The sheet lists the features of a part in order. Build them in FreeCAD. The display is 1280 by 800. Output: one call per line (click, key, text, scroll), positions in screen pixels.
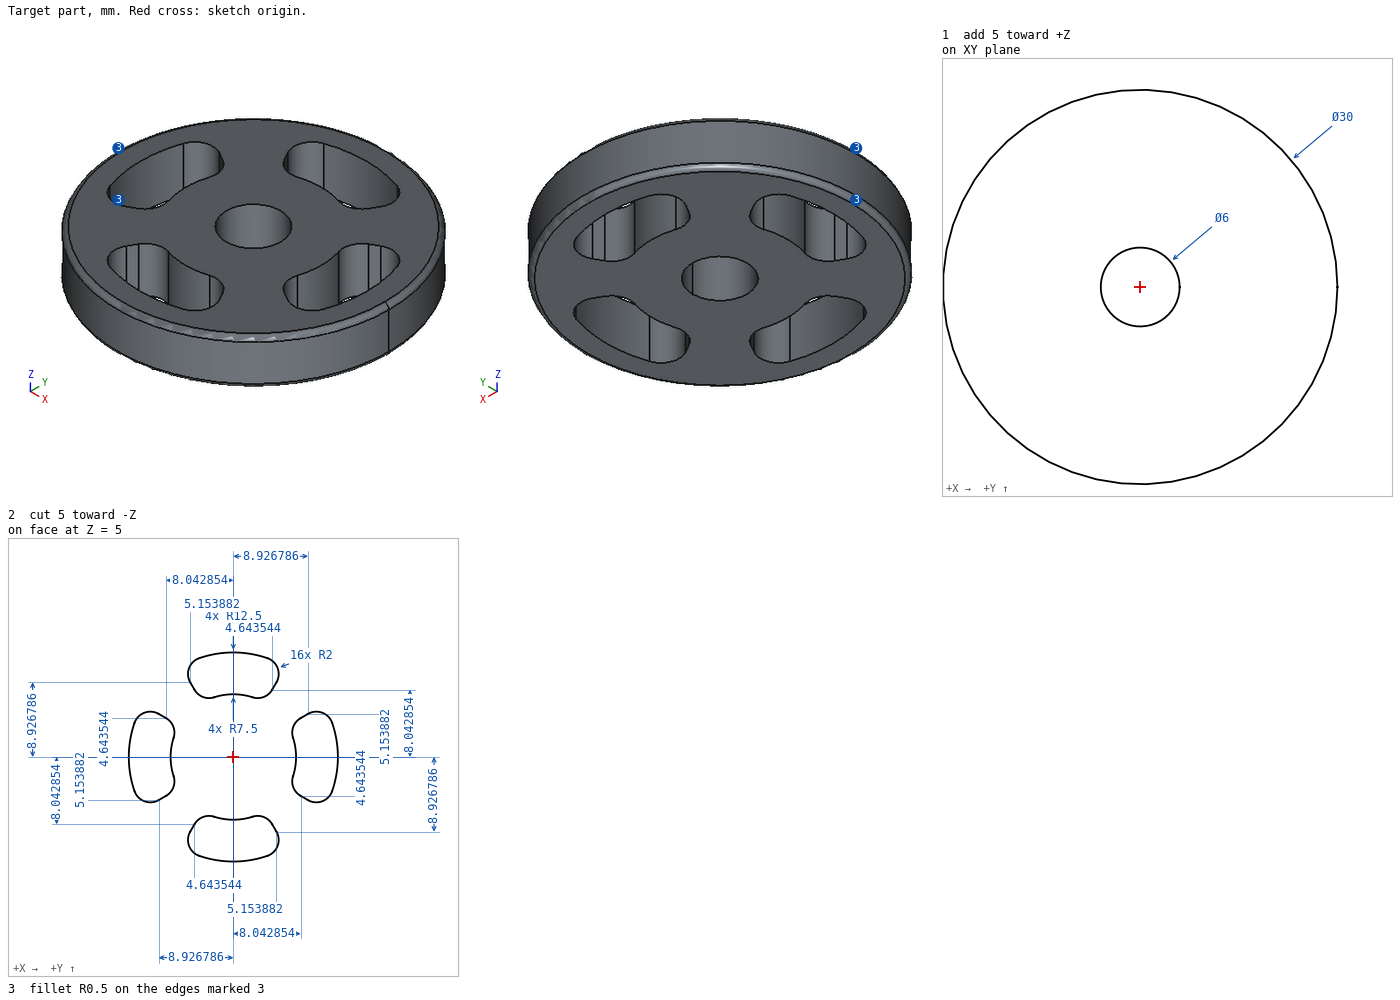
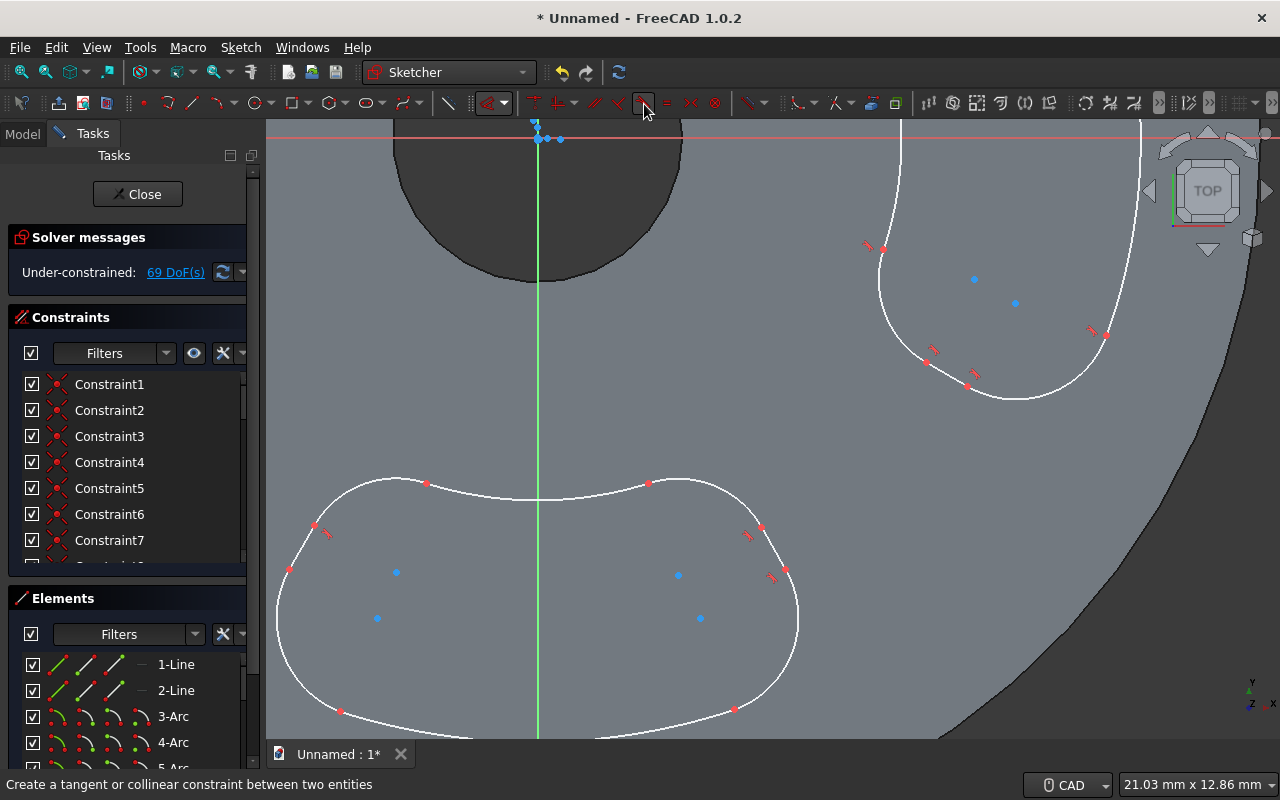
click(307, 539)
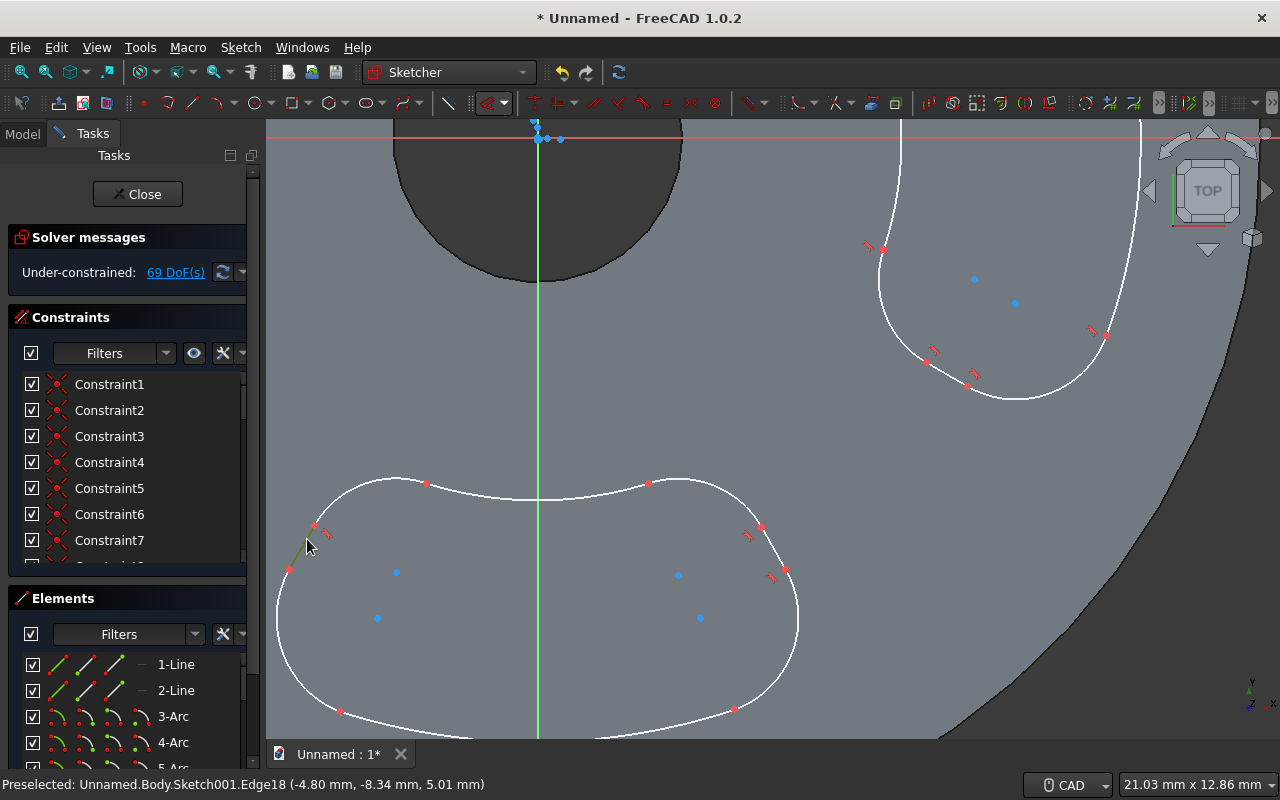
click(299, 682)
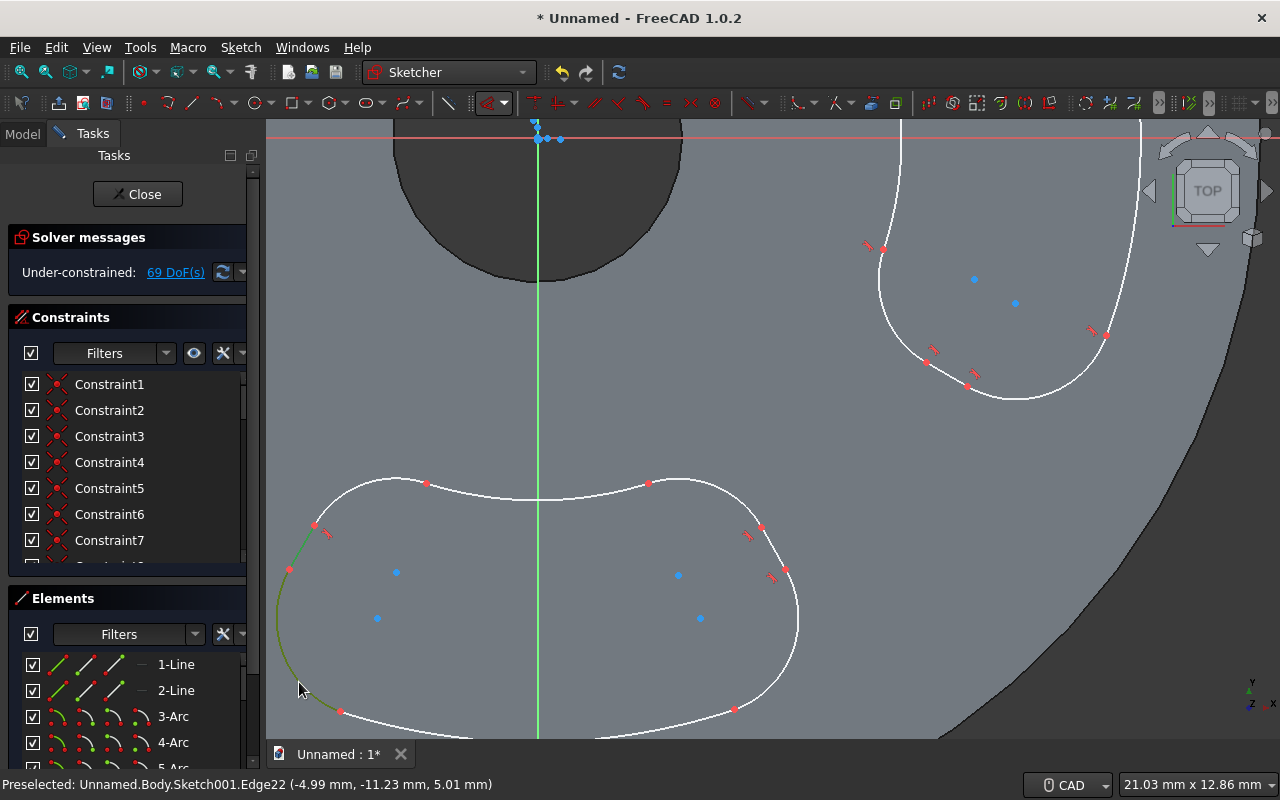
click(644, 104)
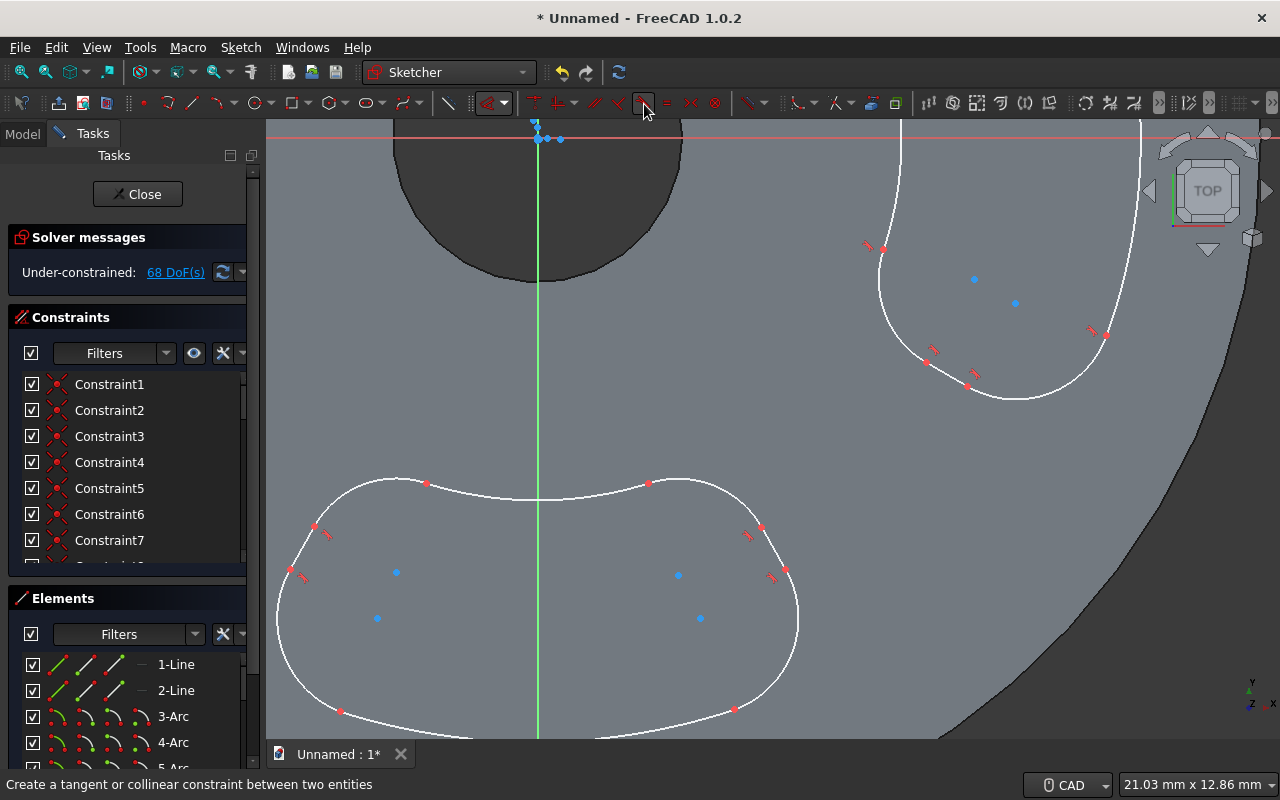
click(736, 498)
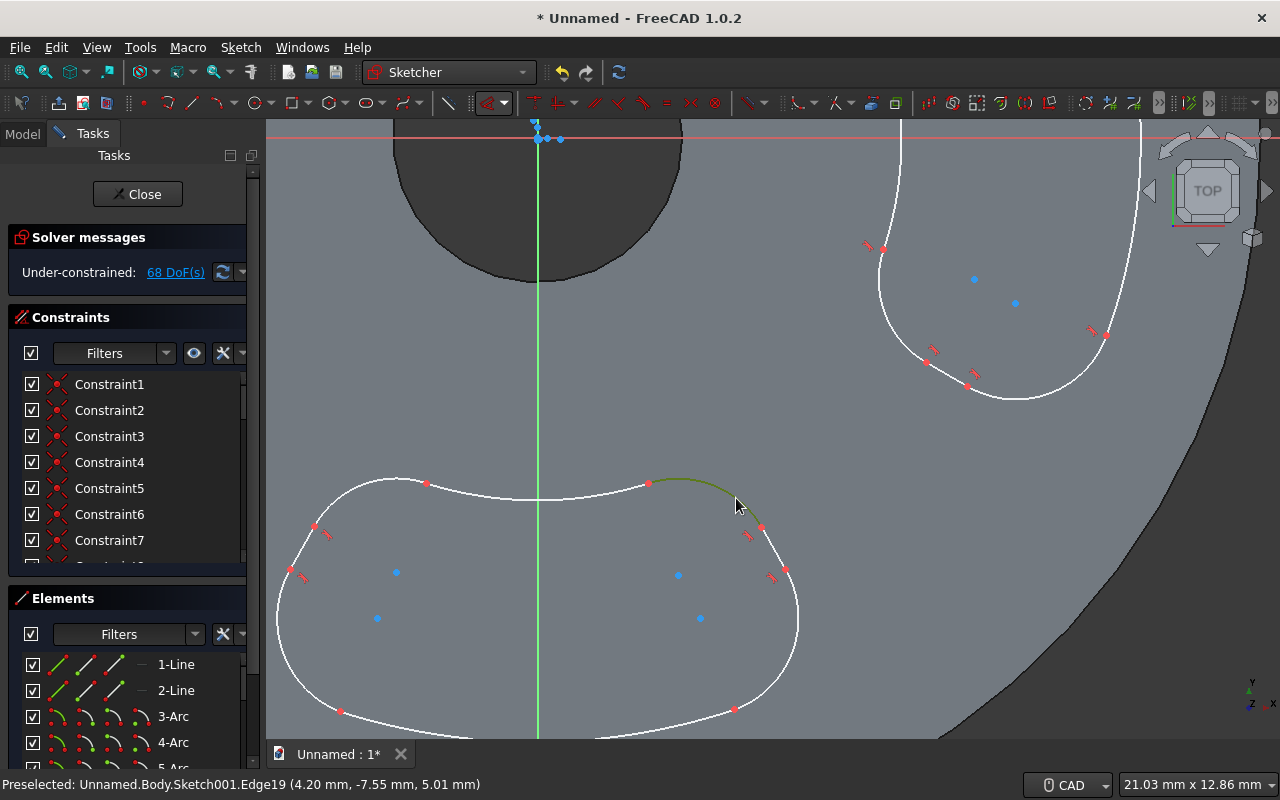
click(492, 498)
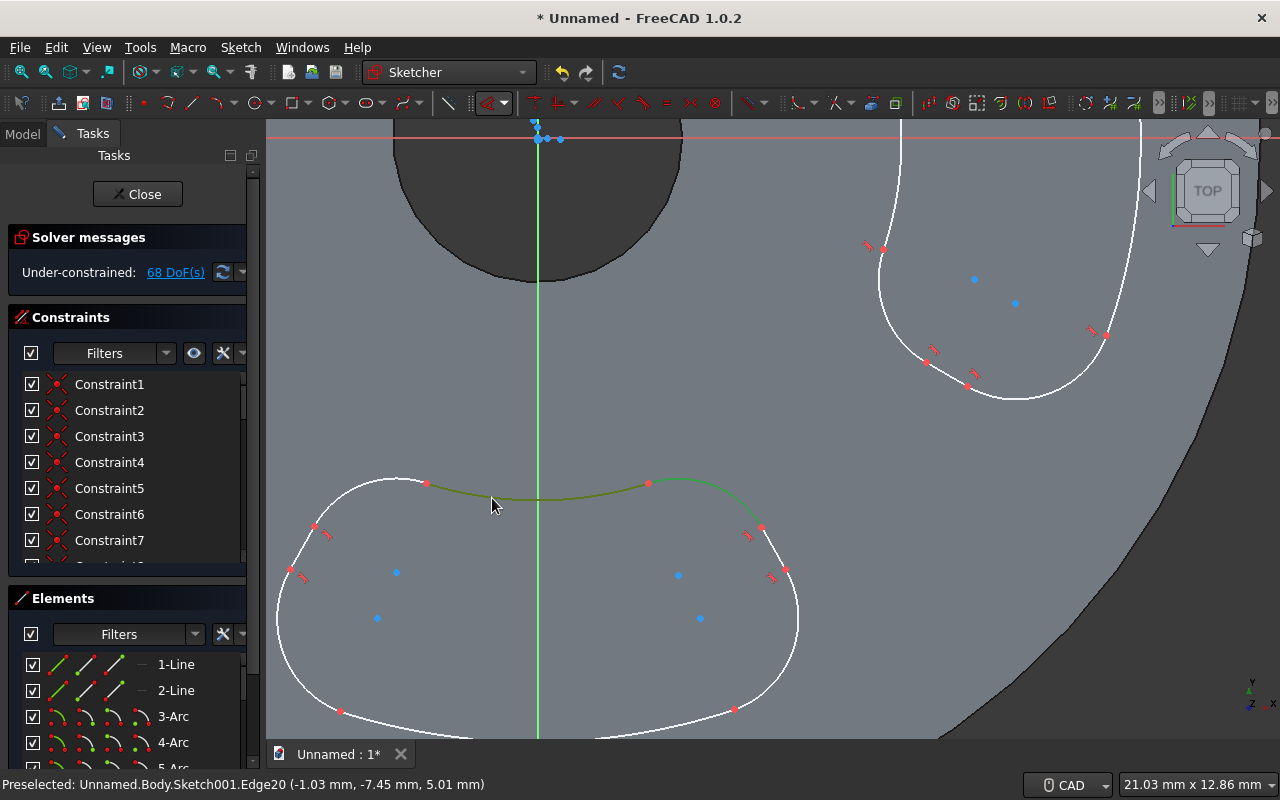
click(644, 104)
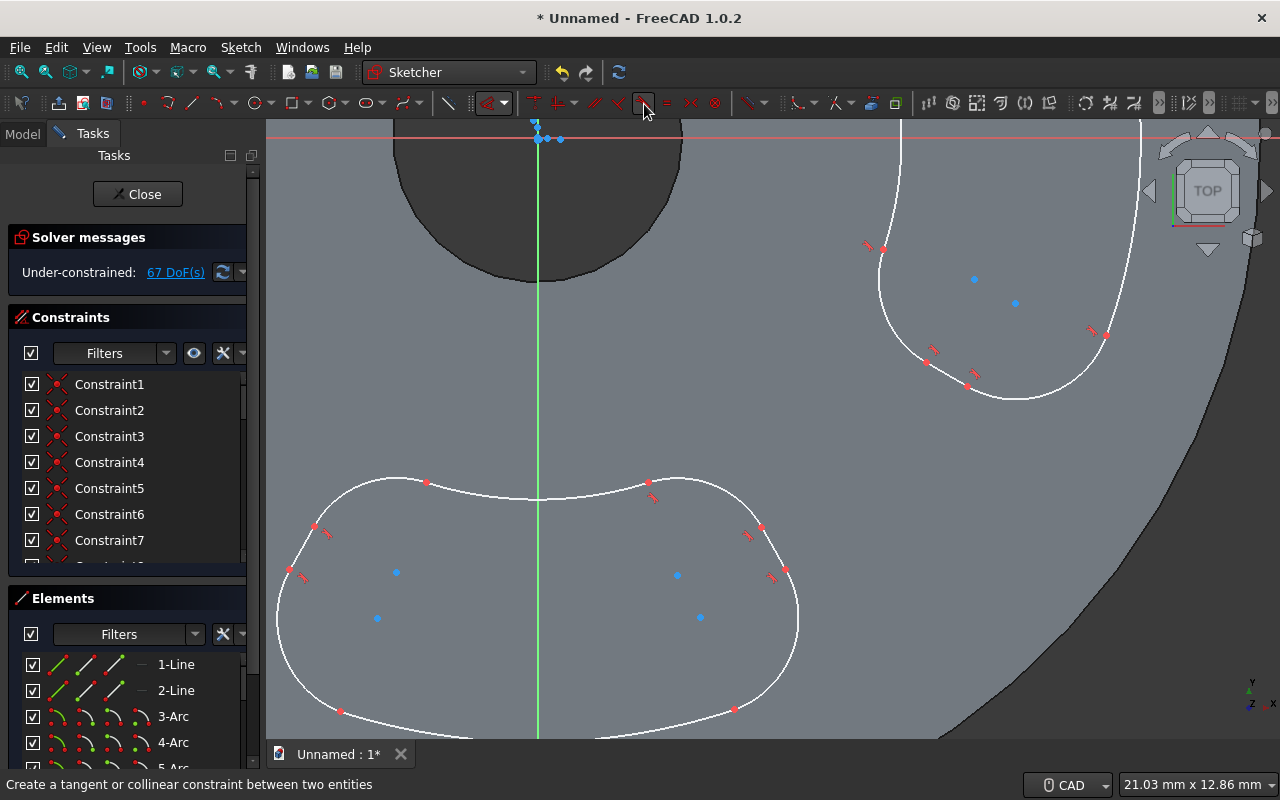
click(492, 497)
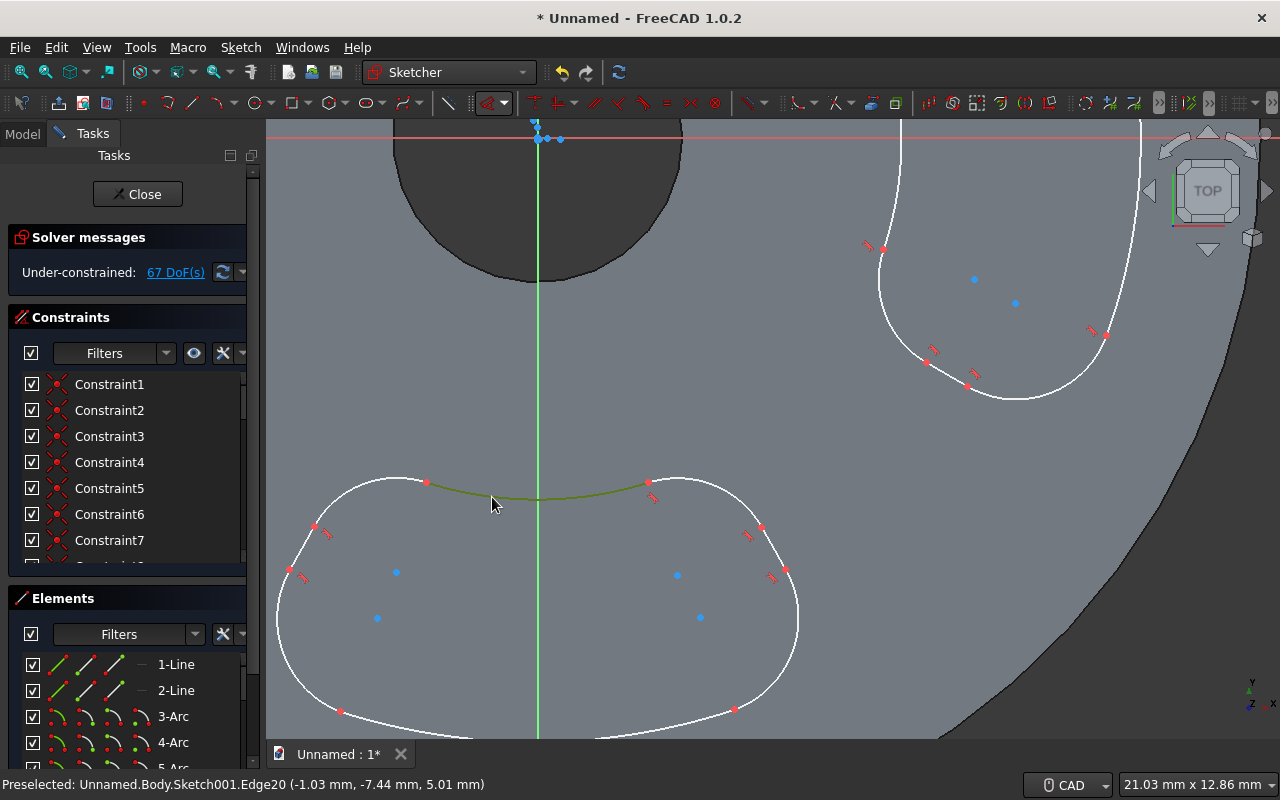
click(388, 478)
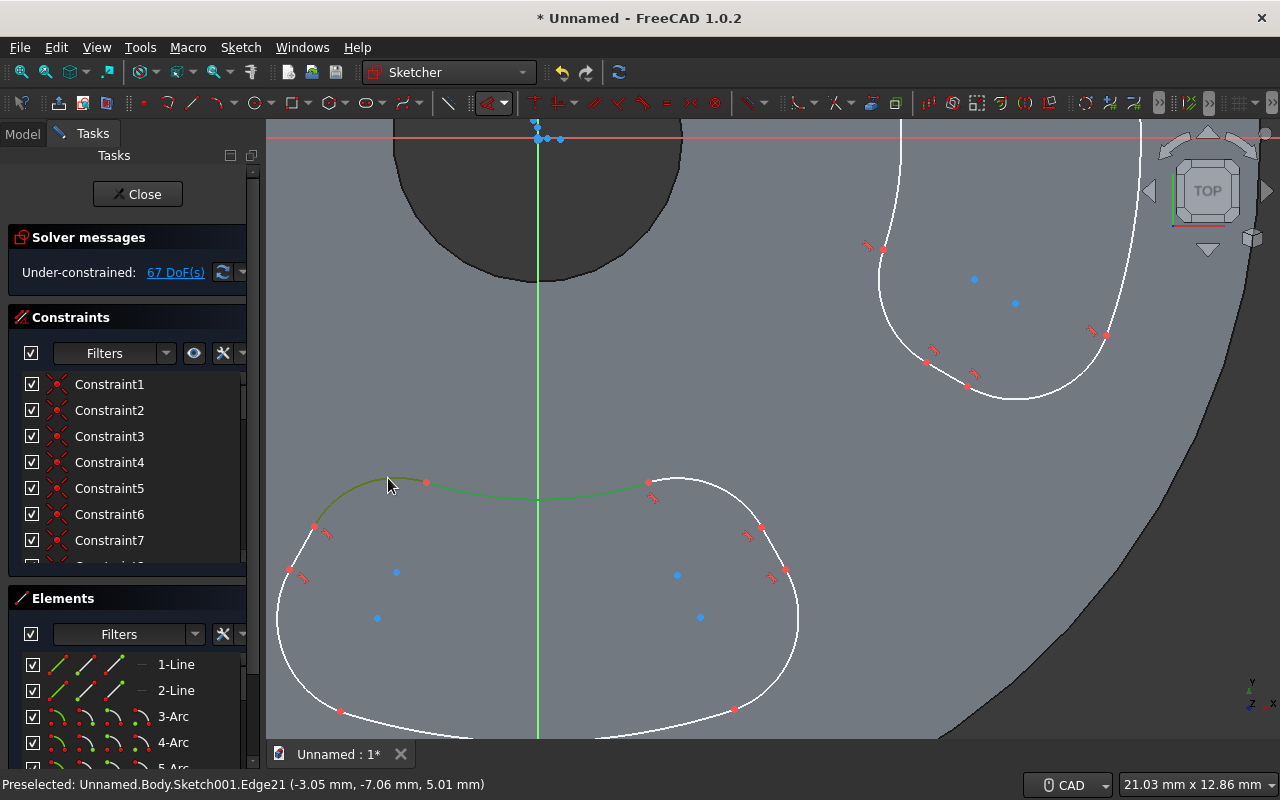
click(644, 104)